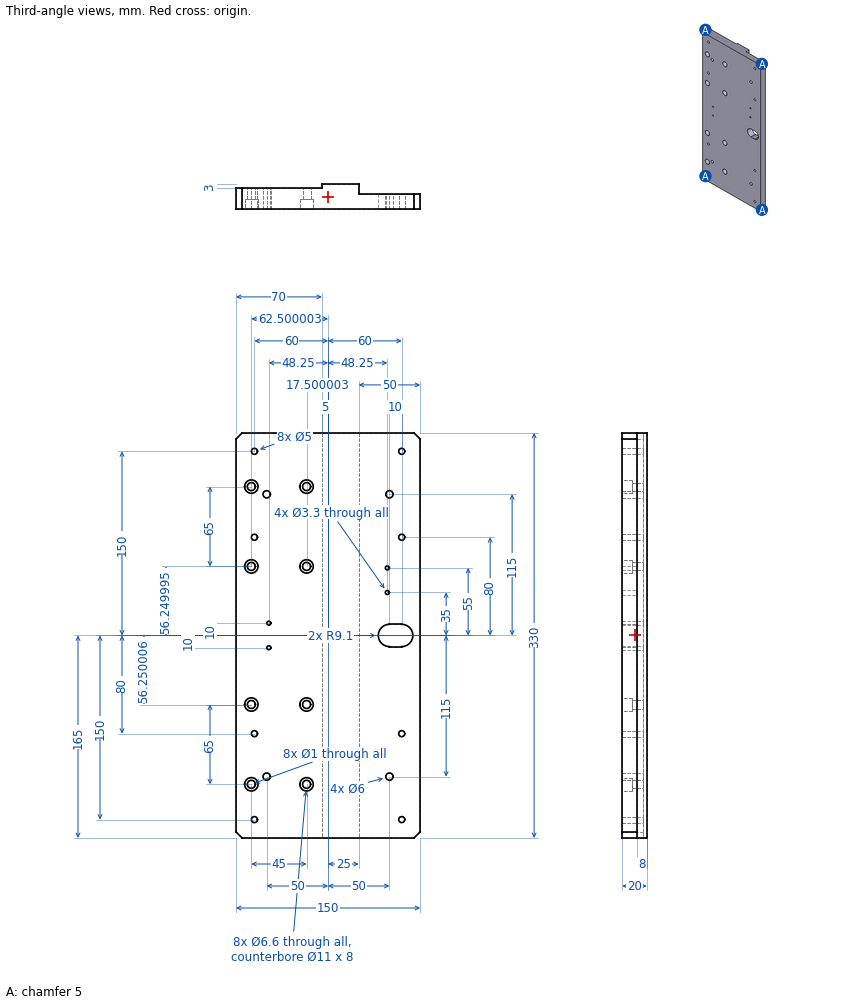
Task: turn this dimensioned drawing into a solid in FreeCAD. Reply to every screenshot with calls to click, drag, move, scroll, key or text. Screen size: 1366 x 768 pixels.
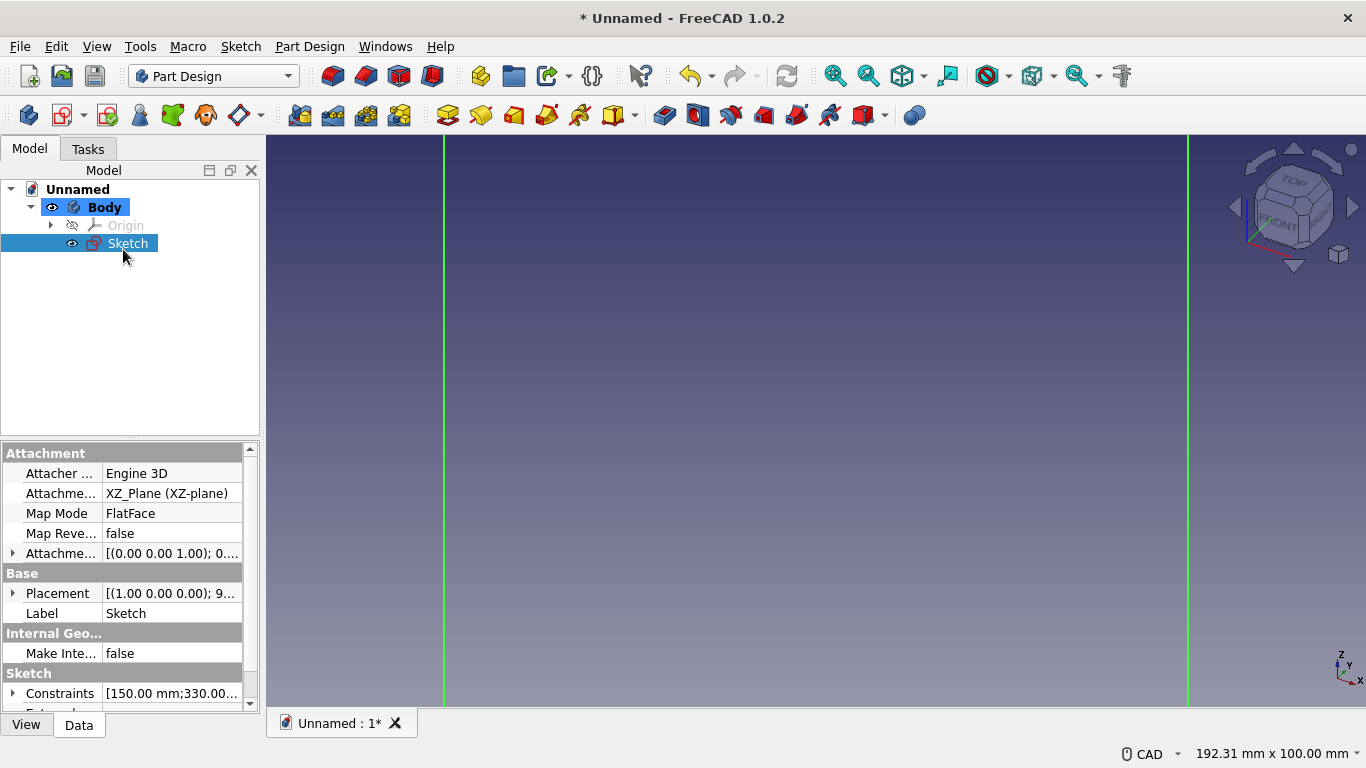
click(448, 116)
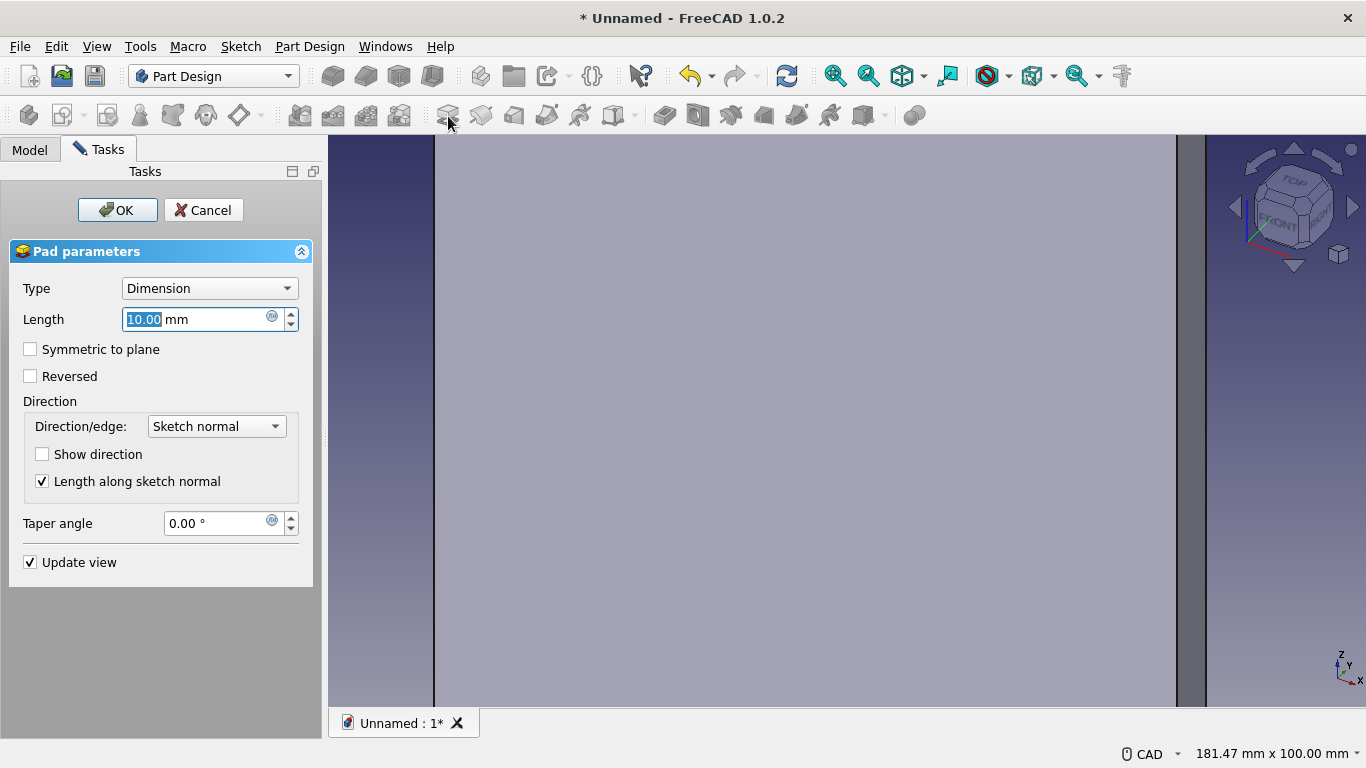
text(20)
key(Tab)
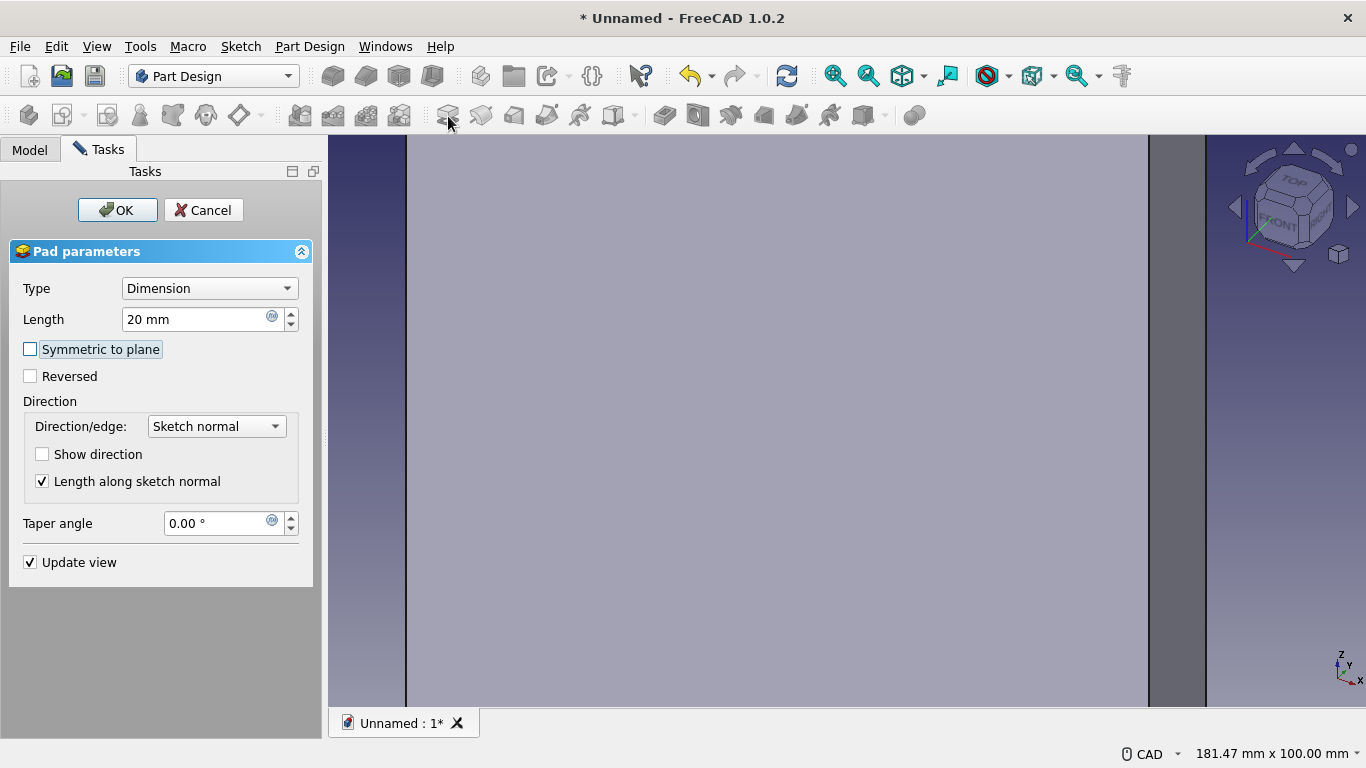
click(31, 349)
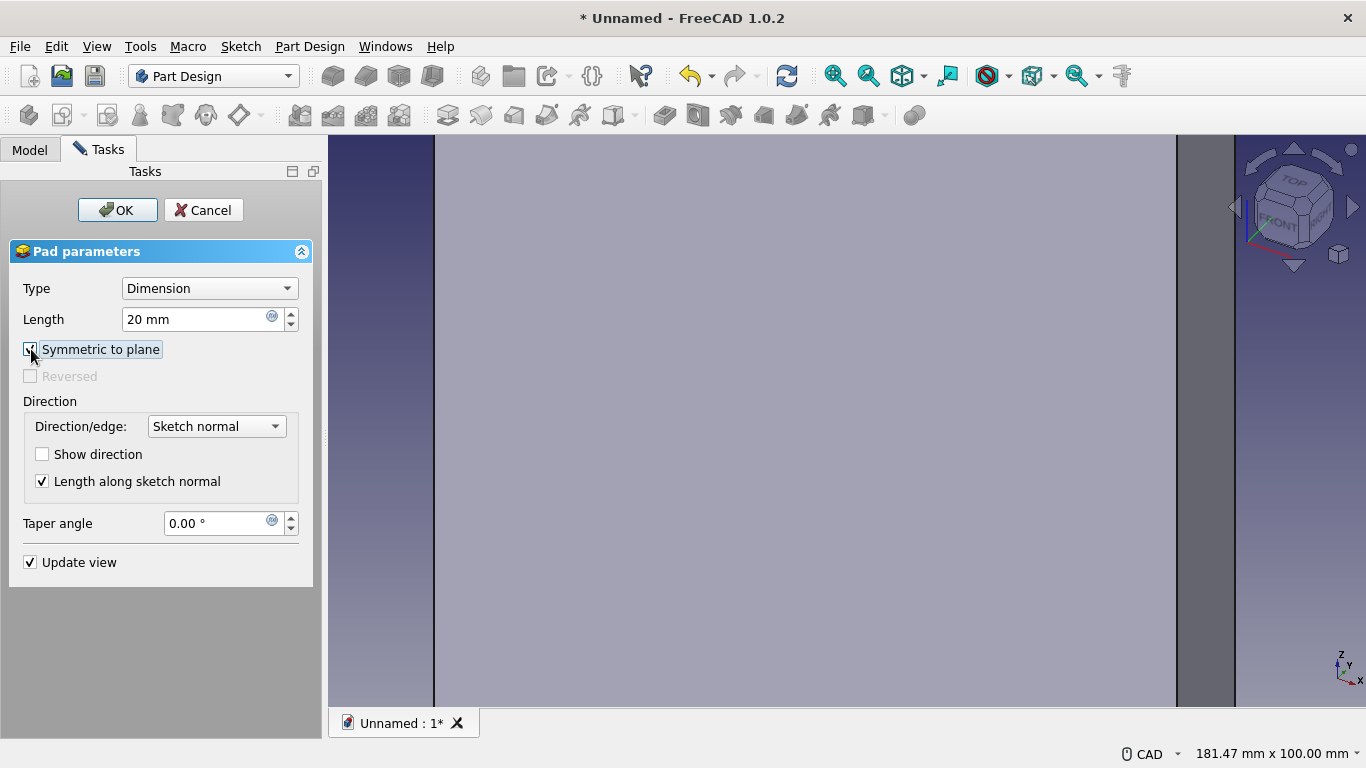
click(118, 210)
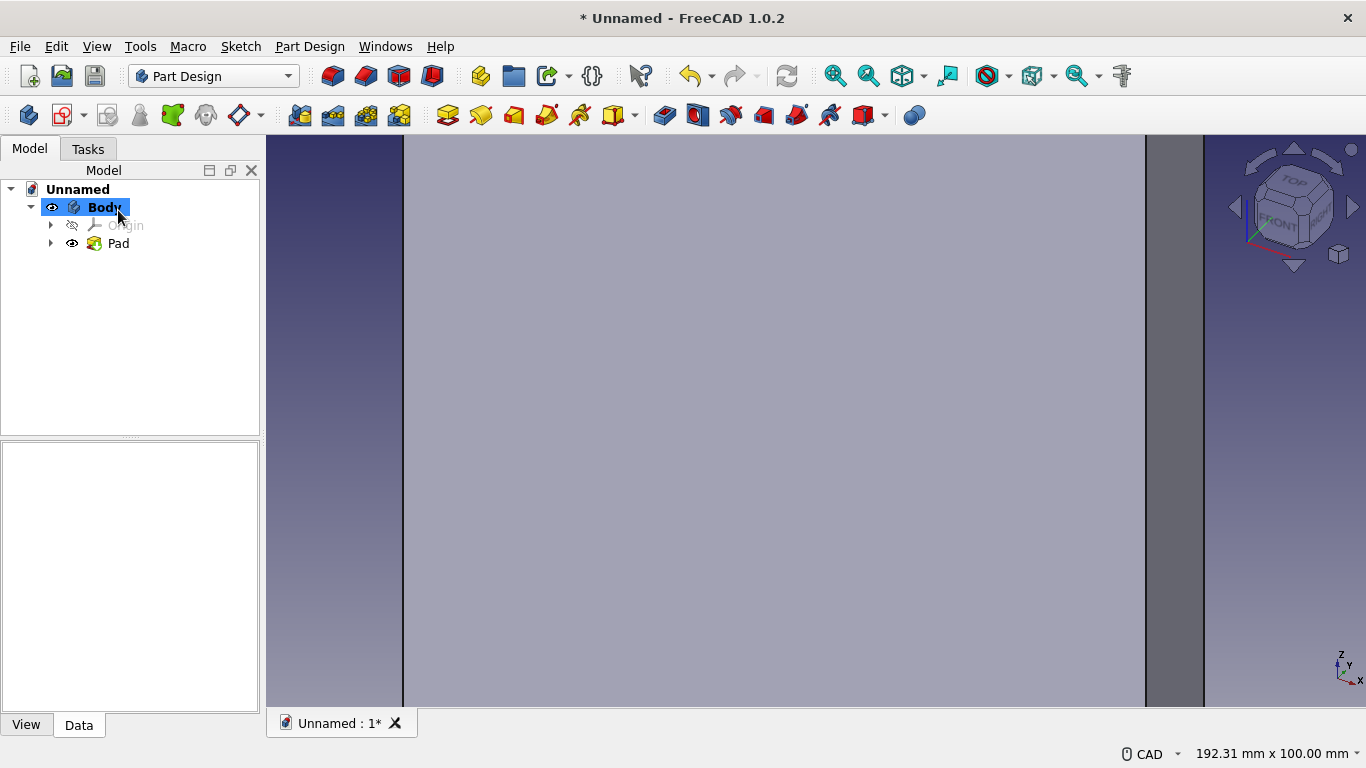
click(836, 76)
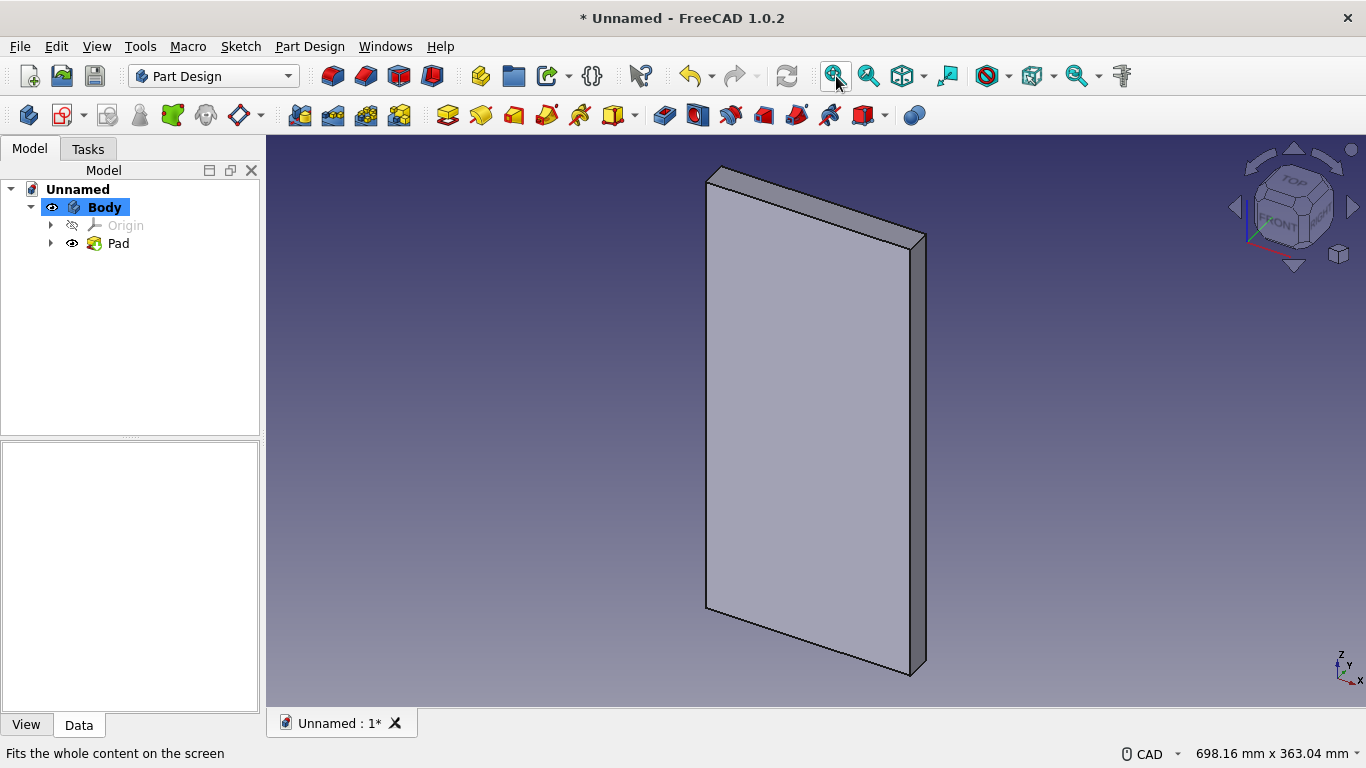
key(4)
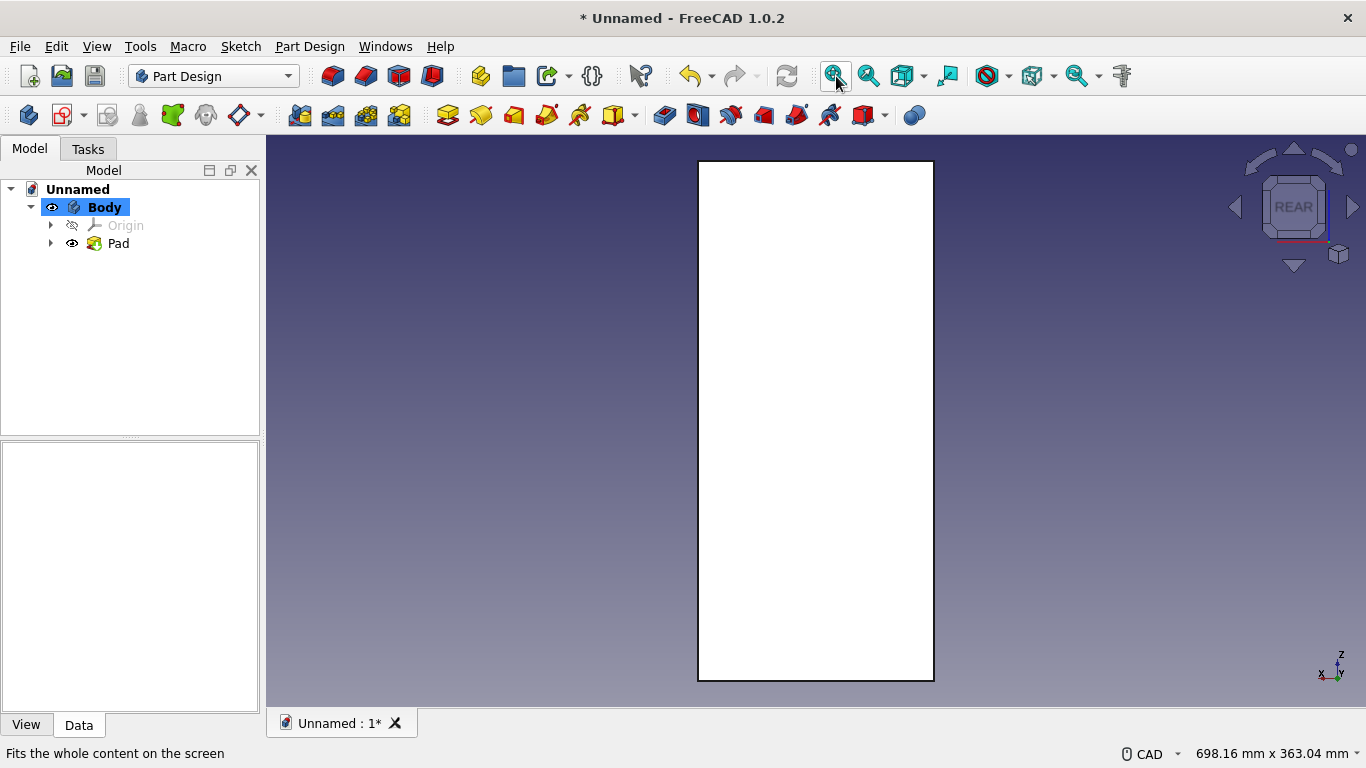
click(816, 346)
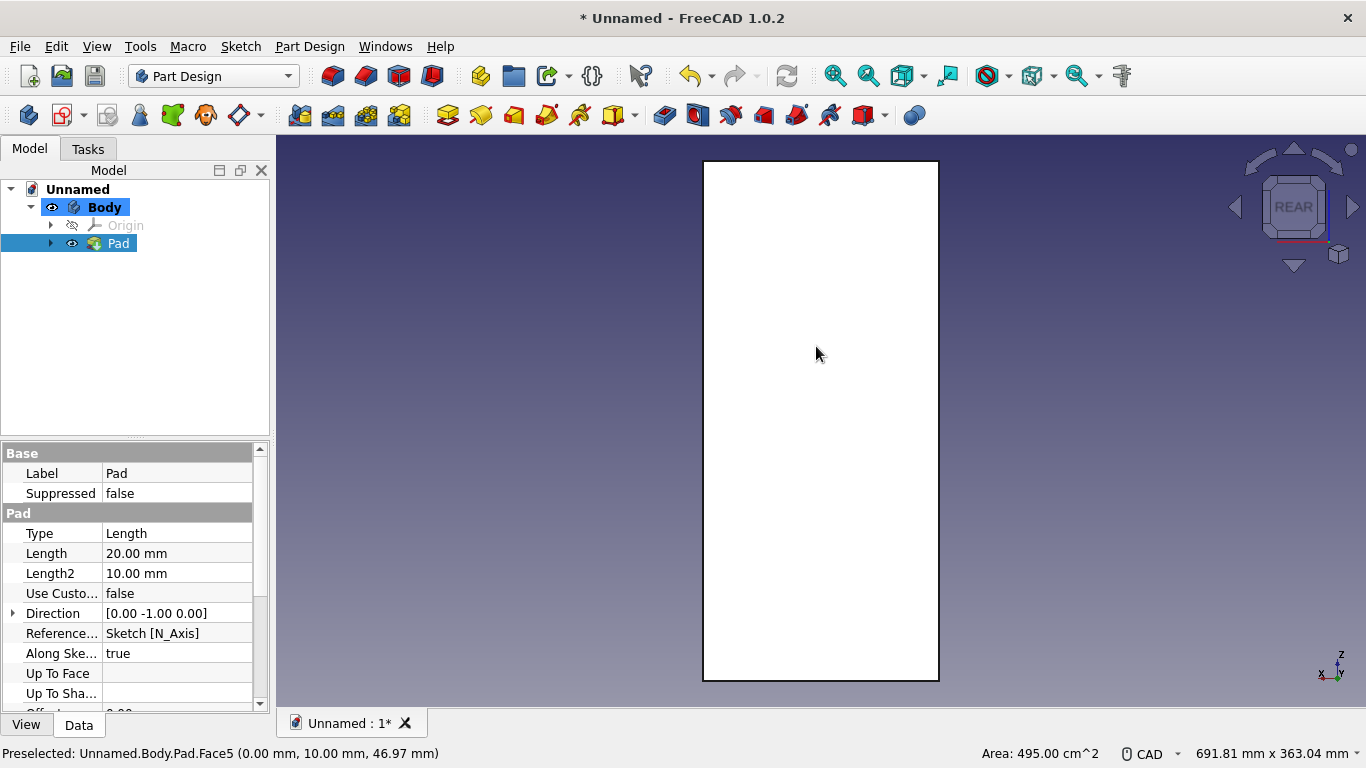
click(62, 116)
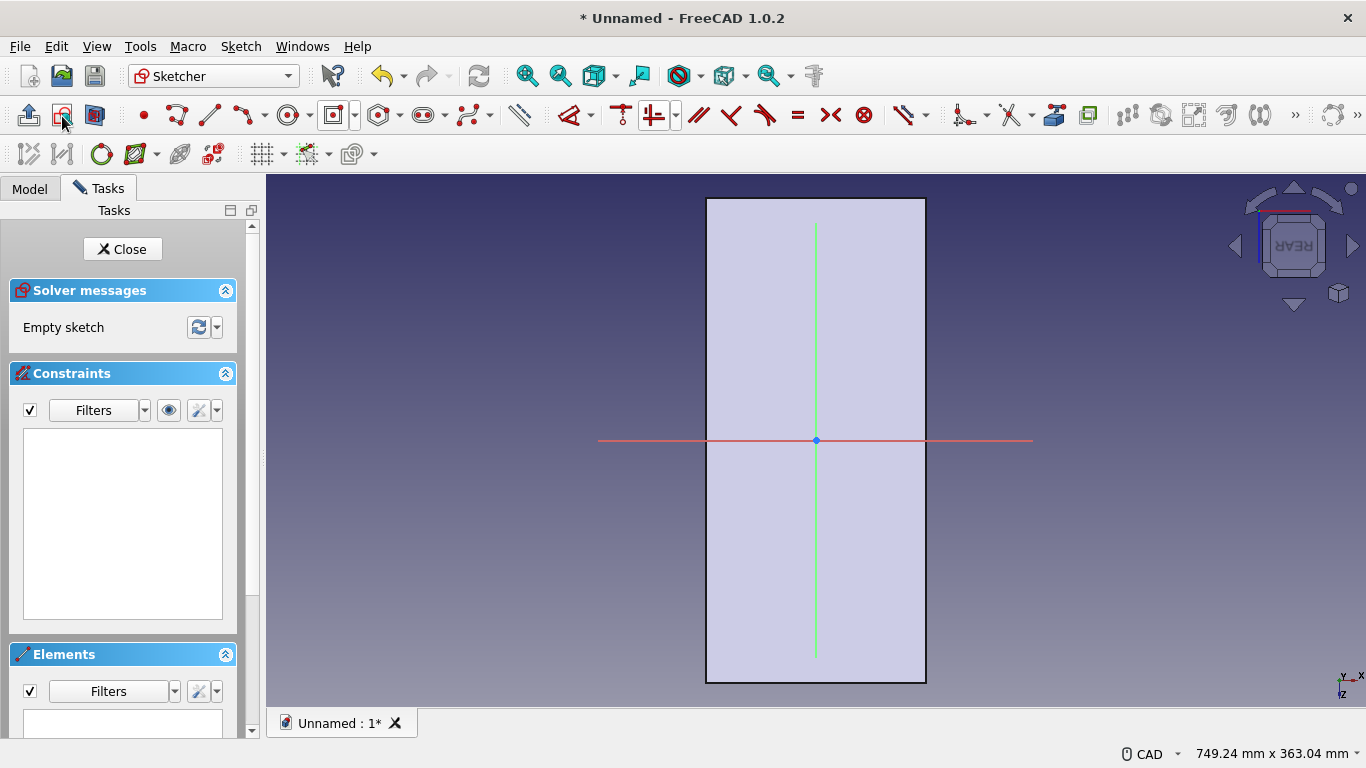
scroll(720, 440, down, 2)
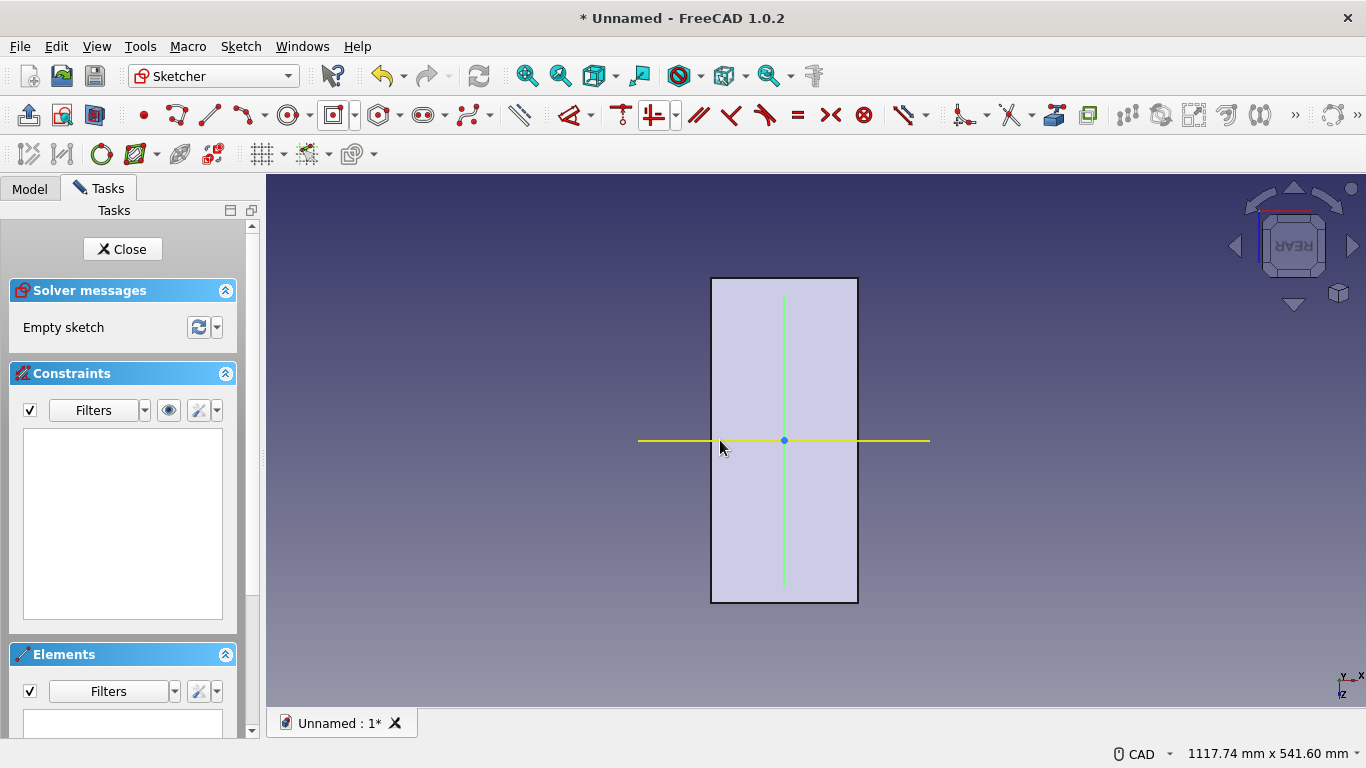
key(g)
key(r)